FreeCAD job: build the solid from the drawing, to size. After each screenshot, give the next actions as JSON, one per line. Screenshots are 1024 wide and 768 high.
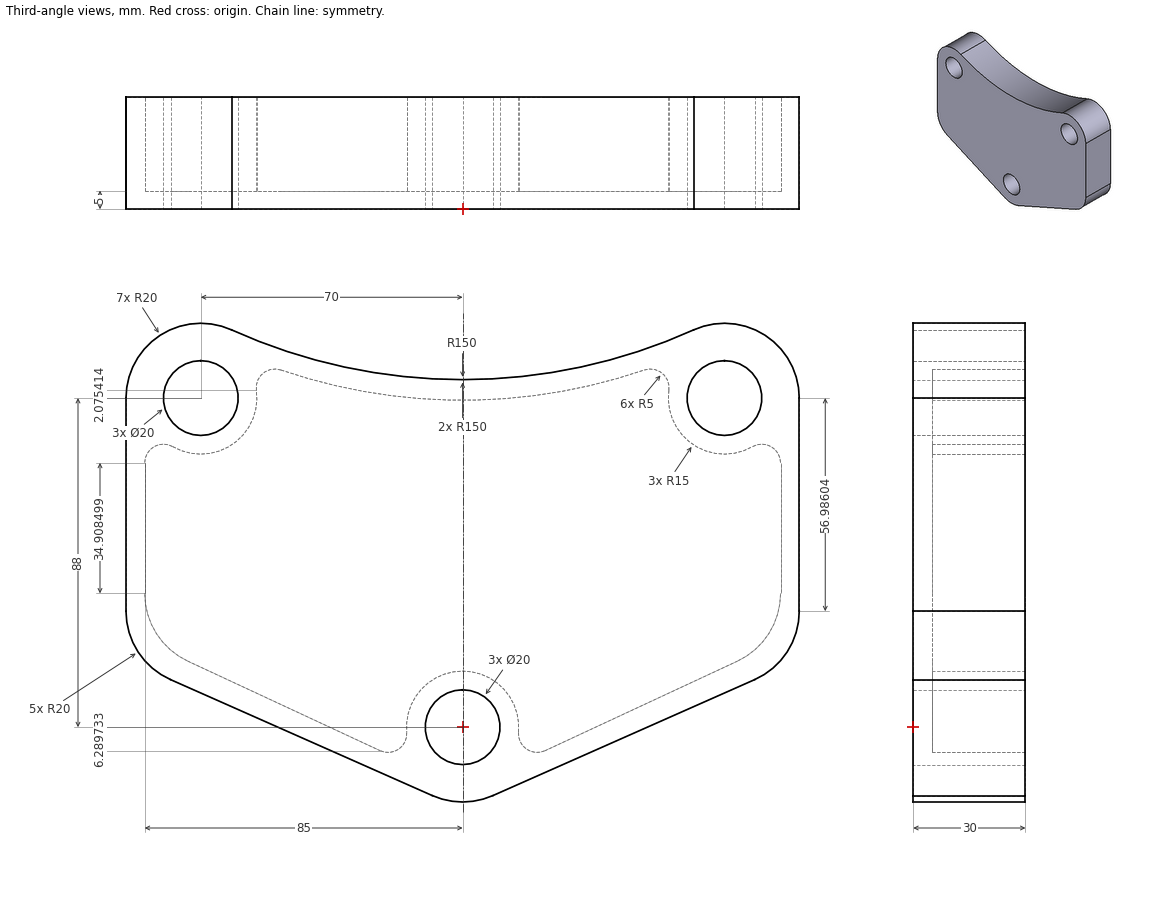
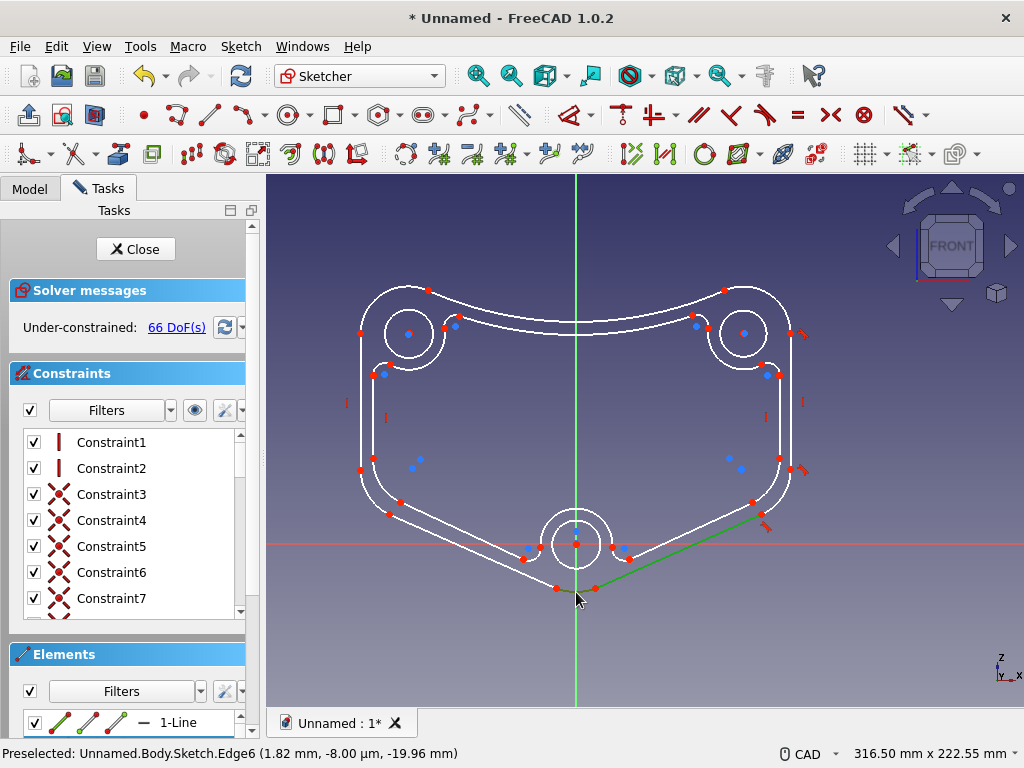
{"action": "left_click", "coordinate": [765, 116]}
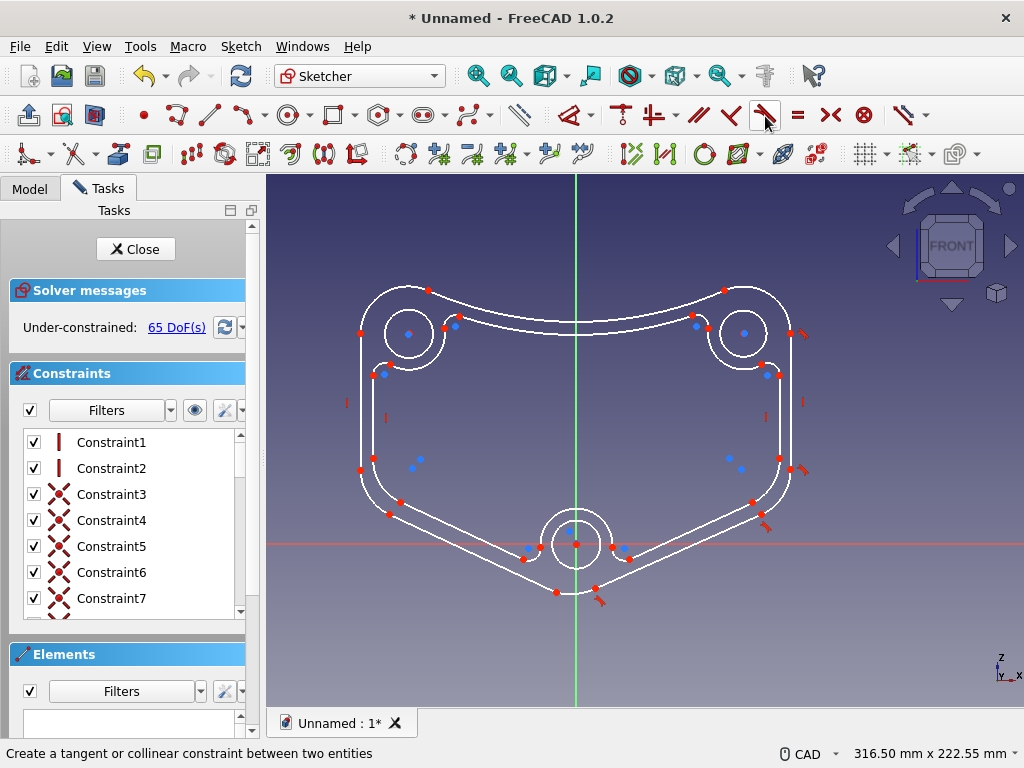
{"action": "left_click", "coordinate": [506, 569]}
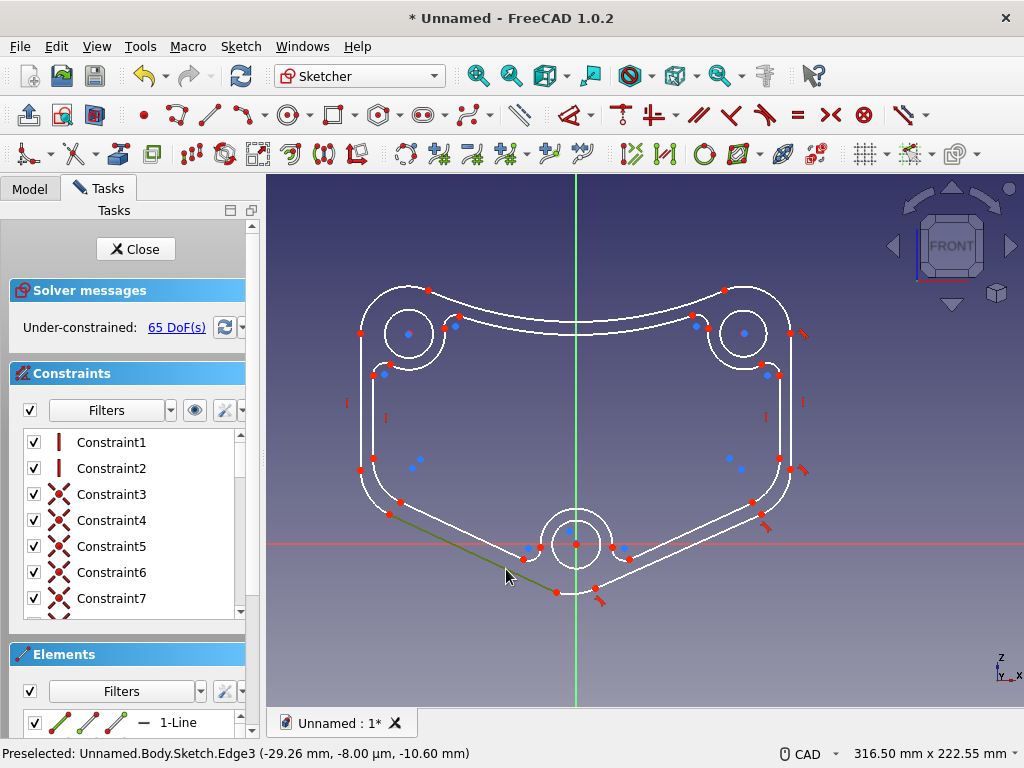
{"action": "left_click", "coordinate": [576, 594]}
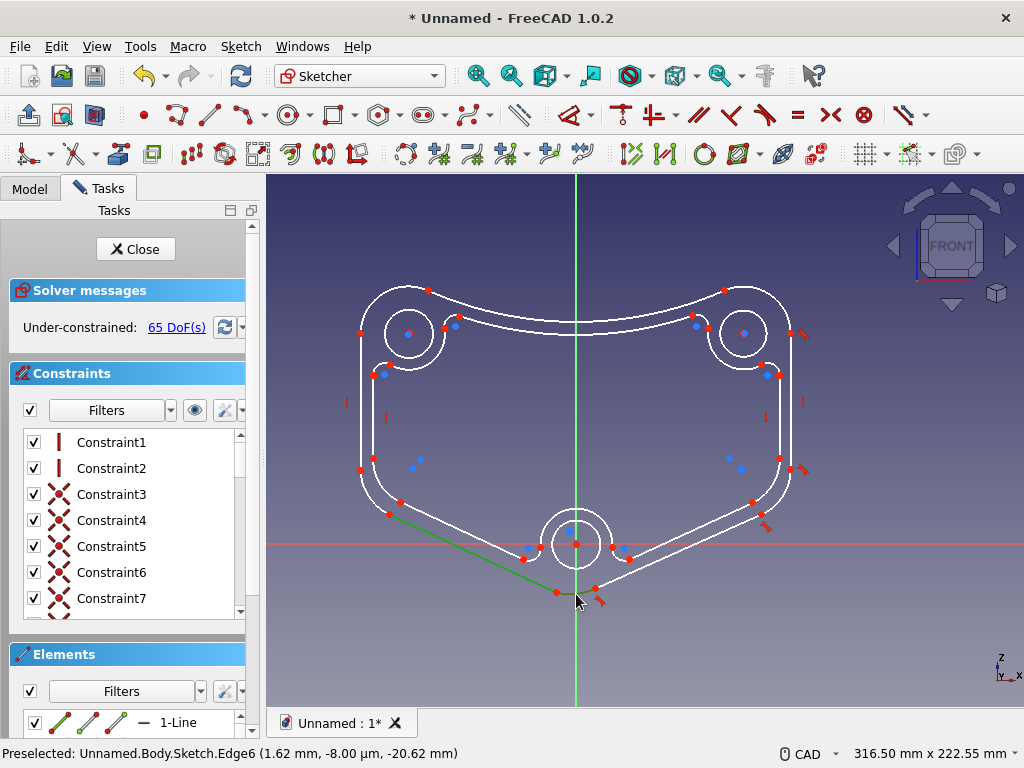
{"action": "left_click", "coordinate": [765, 116]}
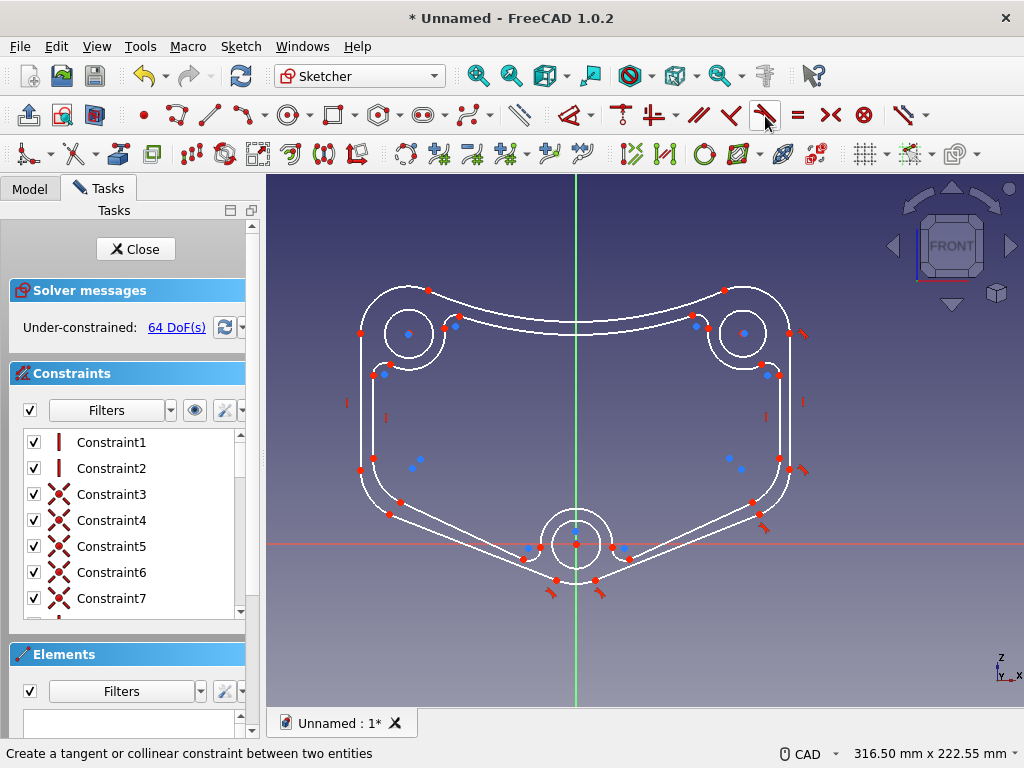
{"action": "scroll", "coordinate": [440, 534], "scroll_direction": "up", "scroll_amount": 2}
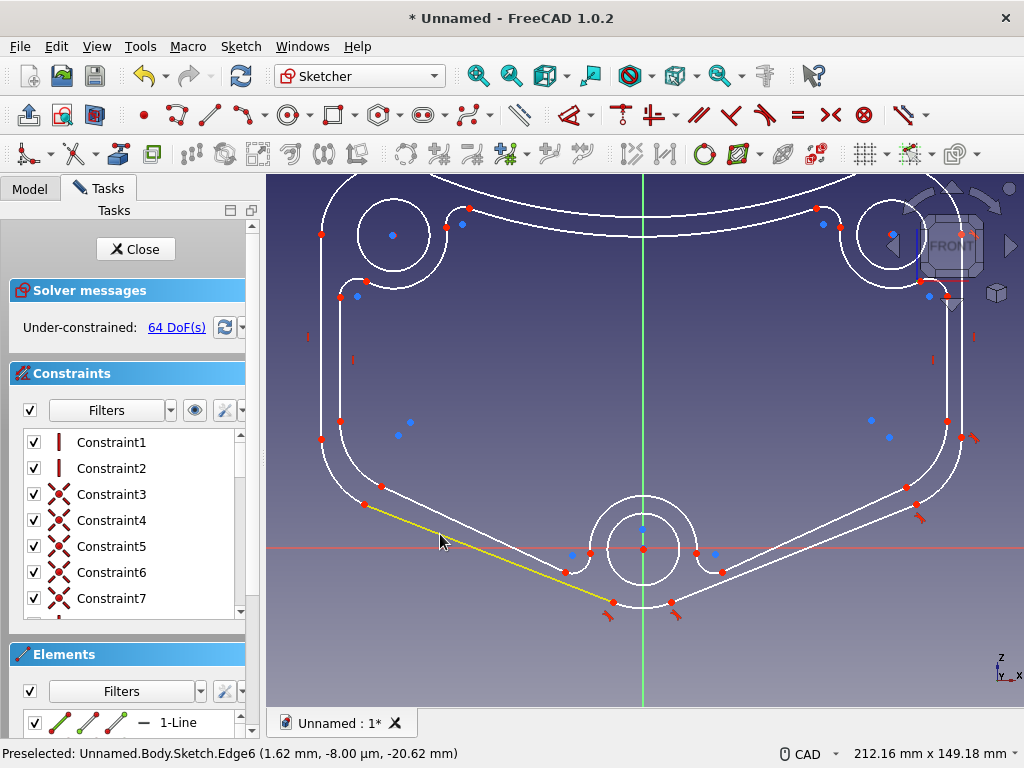
{"action": "left_click", "coordinate": [439, 534]}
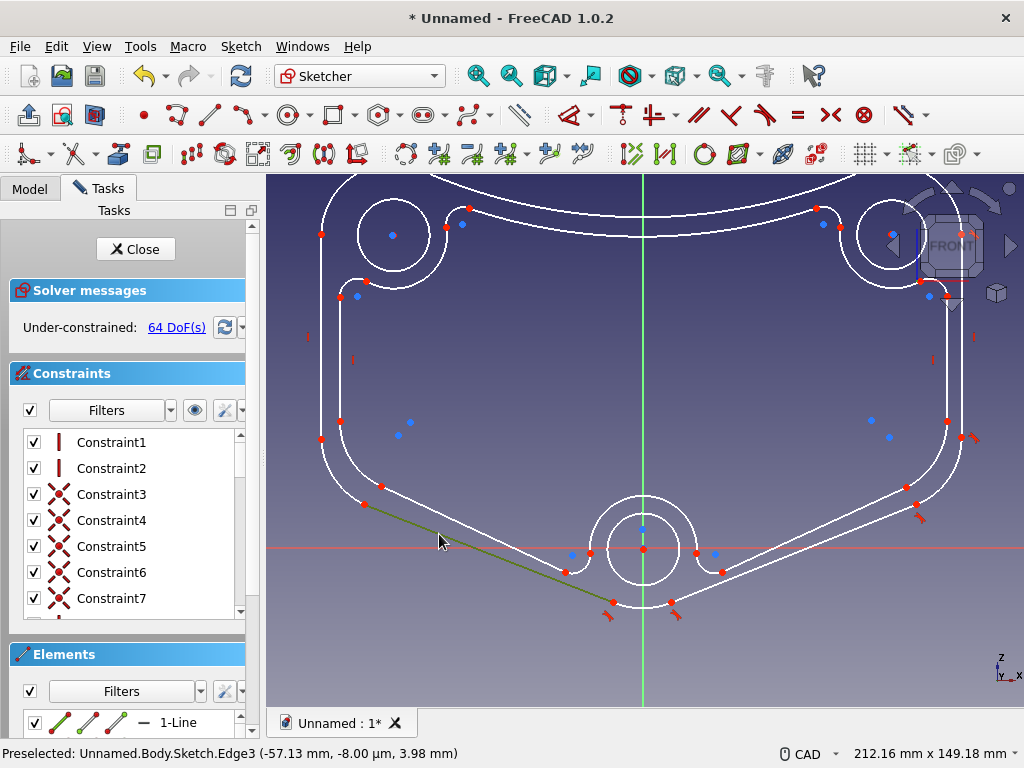
{"action": "left_click", "coordinate": [326, 463]}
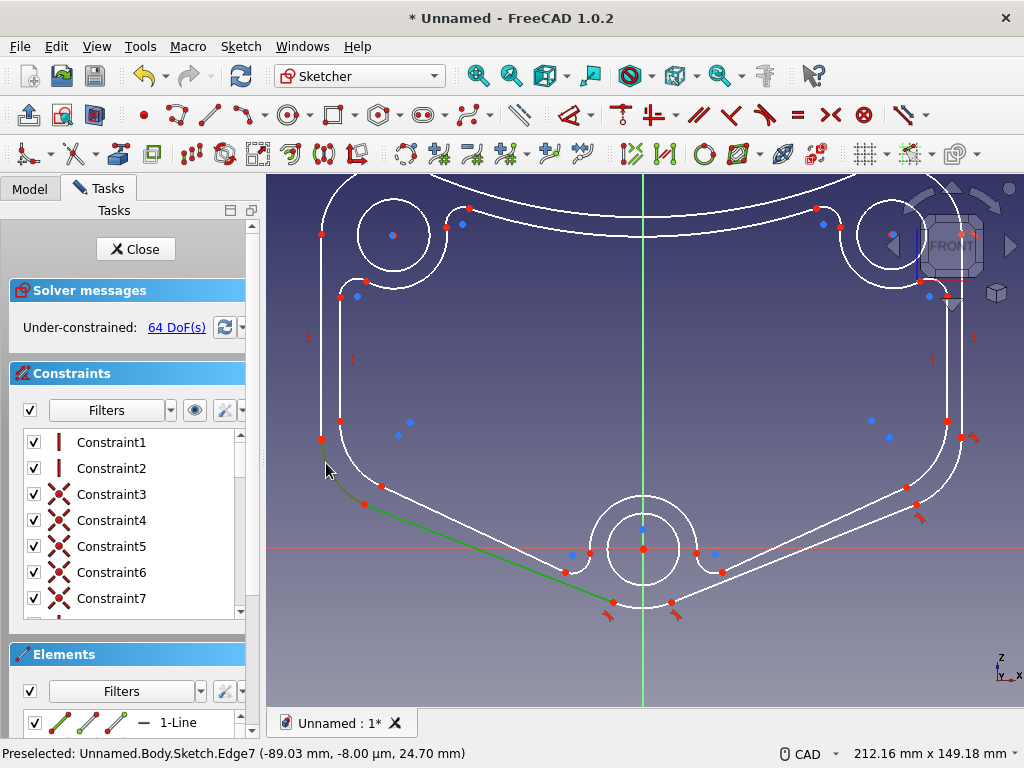
{"action": "left_click", "coordinate": [765, 116]}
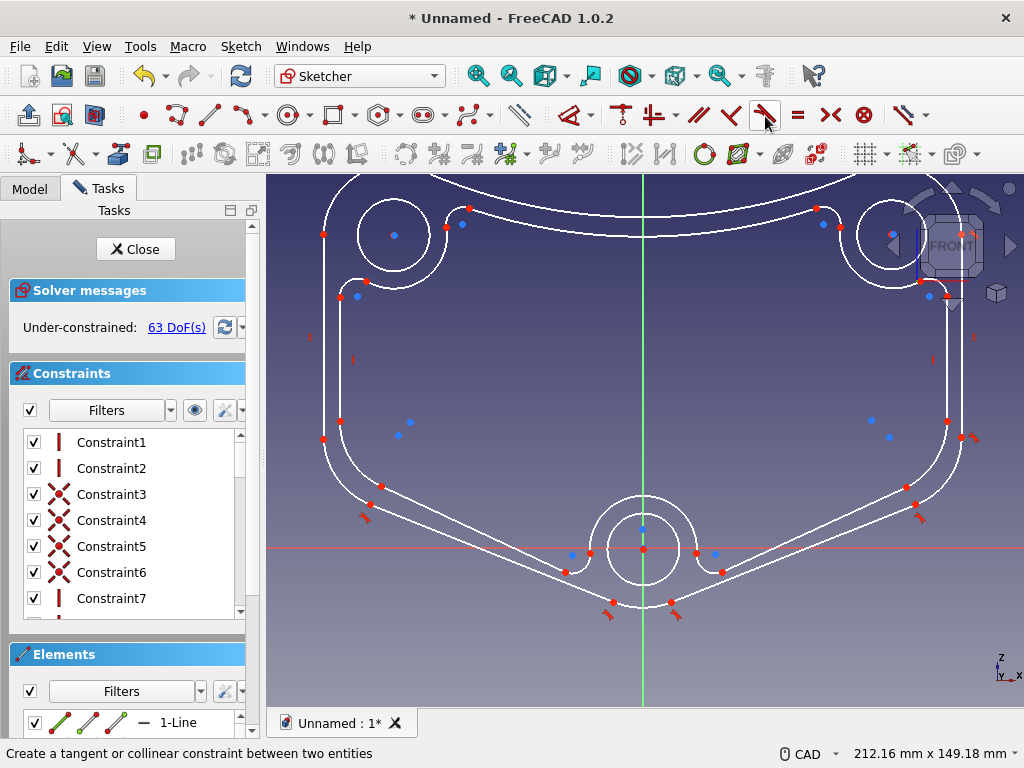
{"action": "left_click", "coordinate": [324, 378]}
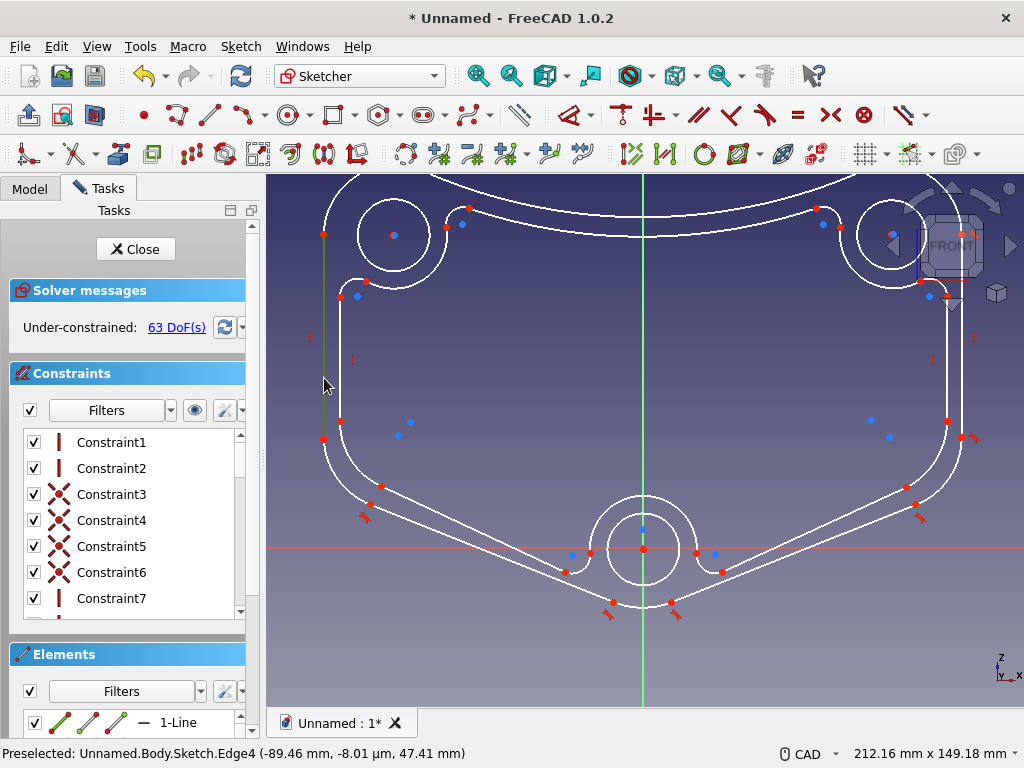
{"action": "left_click", "coordinate": [329, 464]}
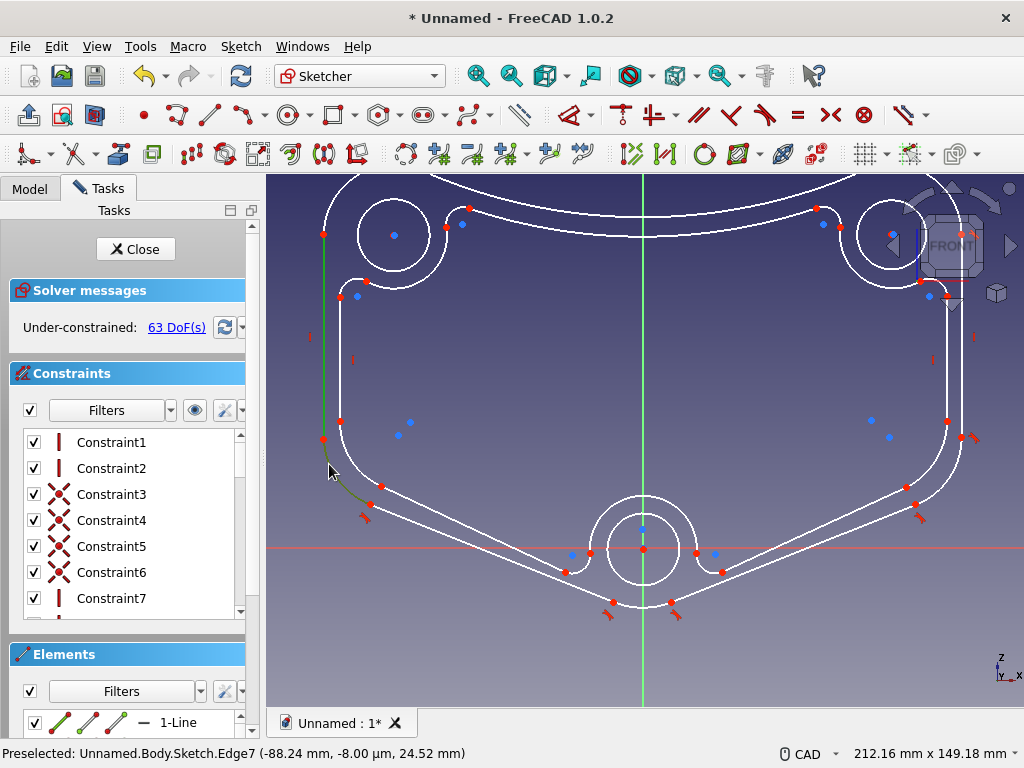
{"action": "left_click", "coordinate": [765, 116]}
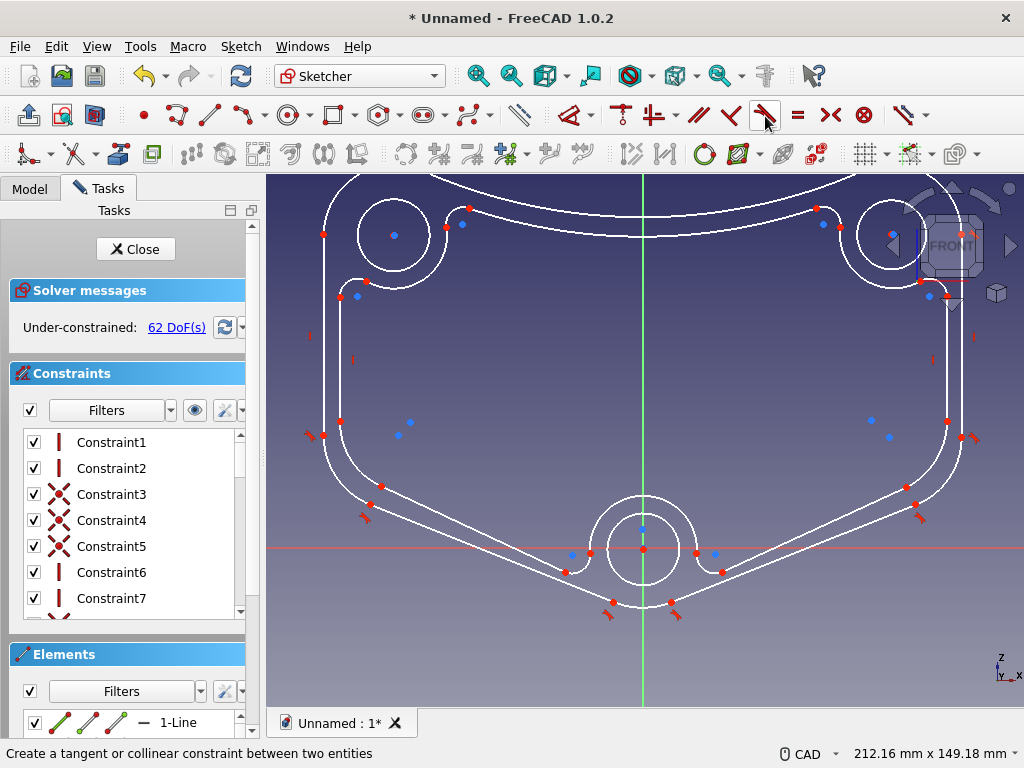
{"action": "left_click", "coordinate": [324, 375]}